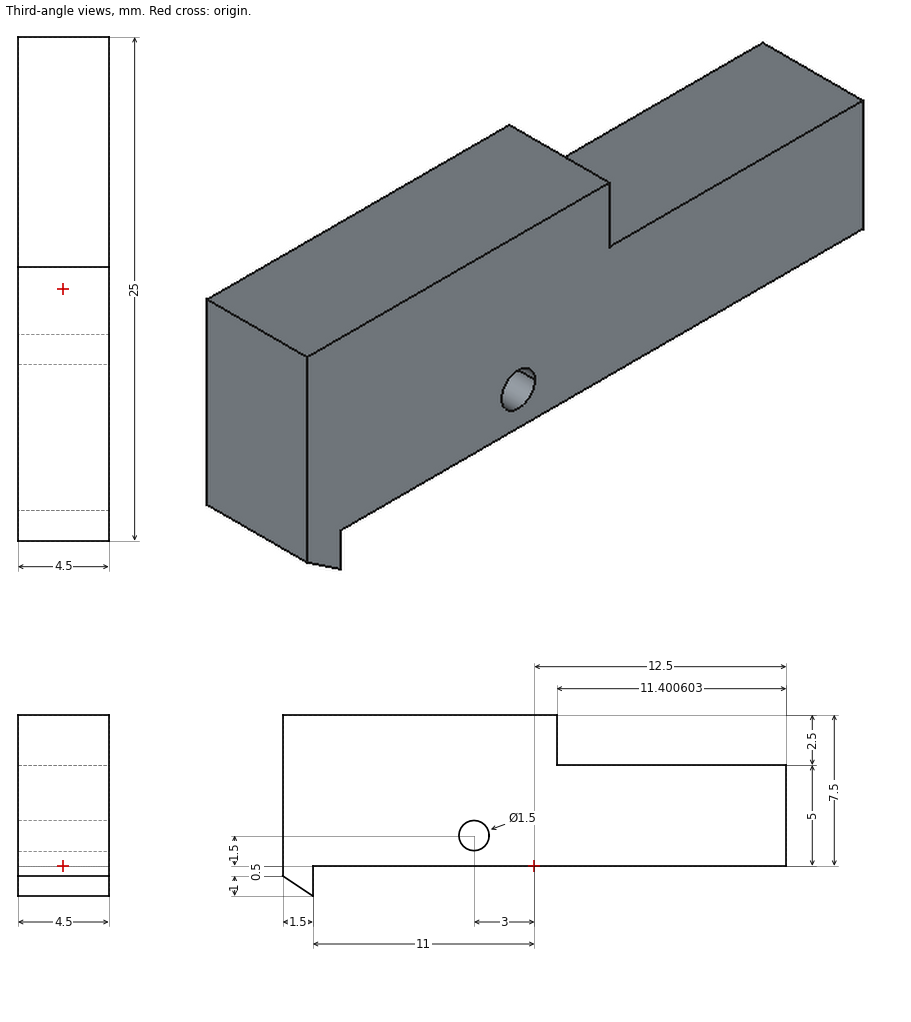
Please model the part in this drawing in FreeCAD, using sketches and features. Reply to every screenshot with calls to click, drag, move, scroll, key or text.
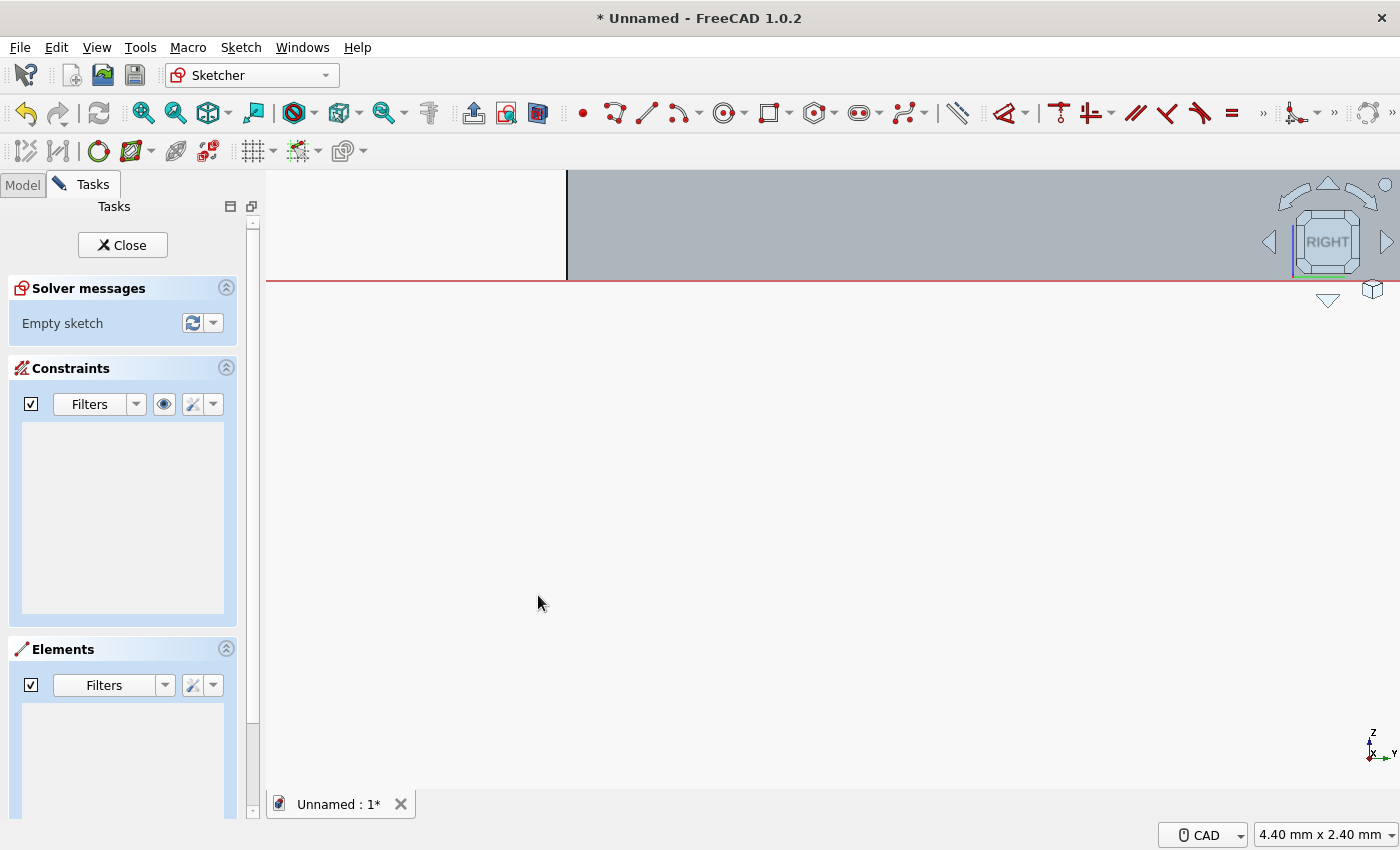
key(g)
key(m)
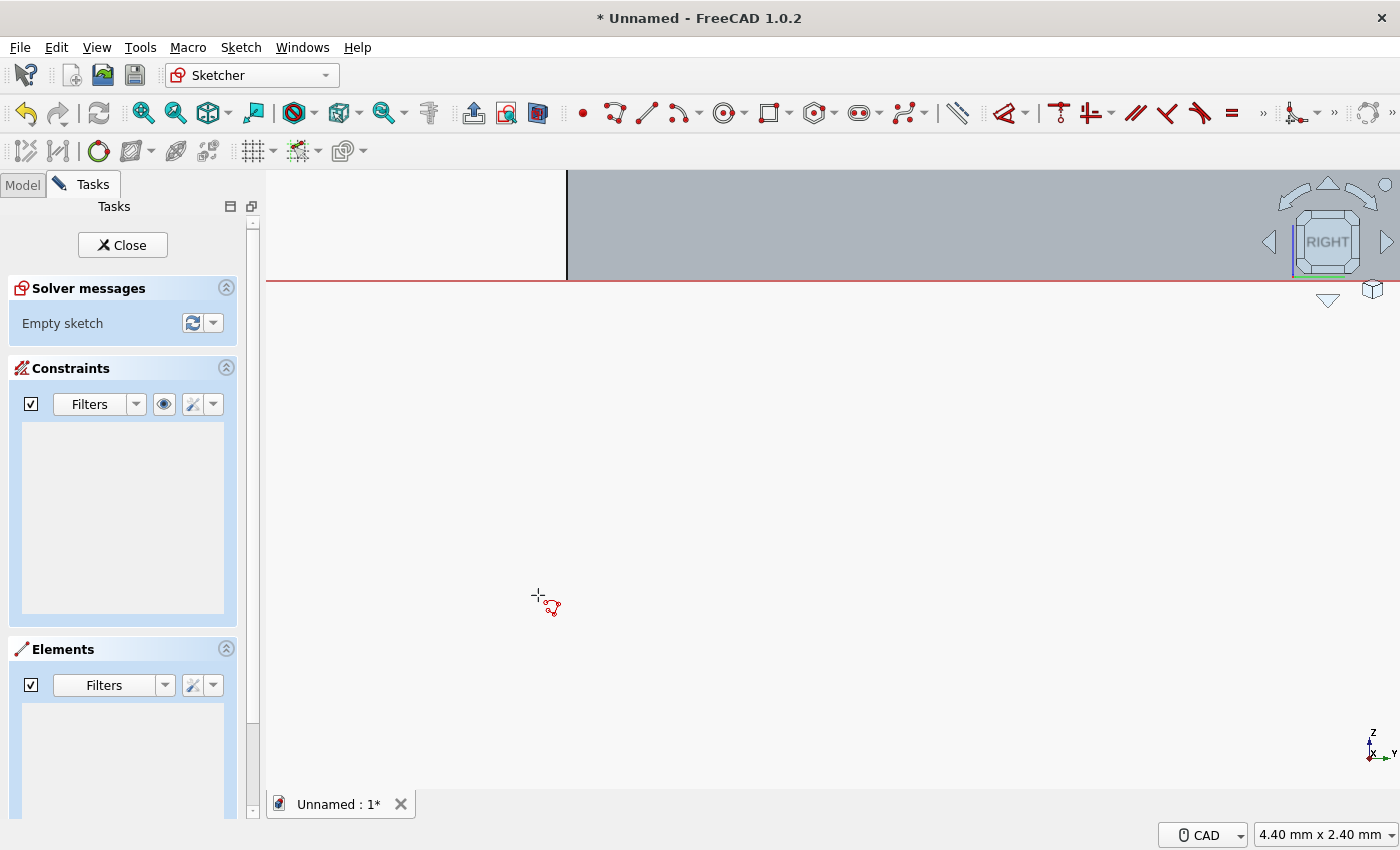
click(954, 281)
click(567, 290)
click(567, 410)
click(954, 667)
click(954, 281)
key(Escape)
key(Escape)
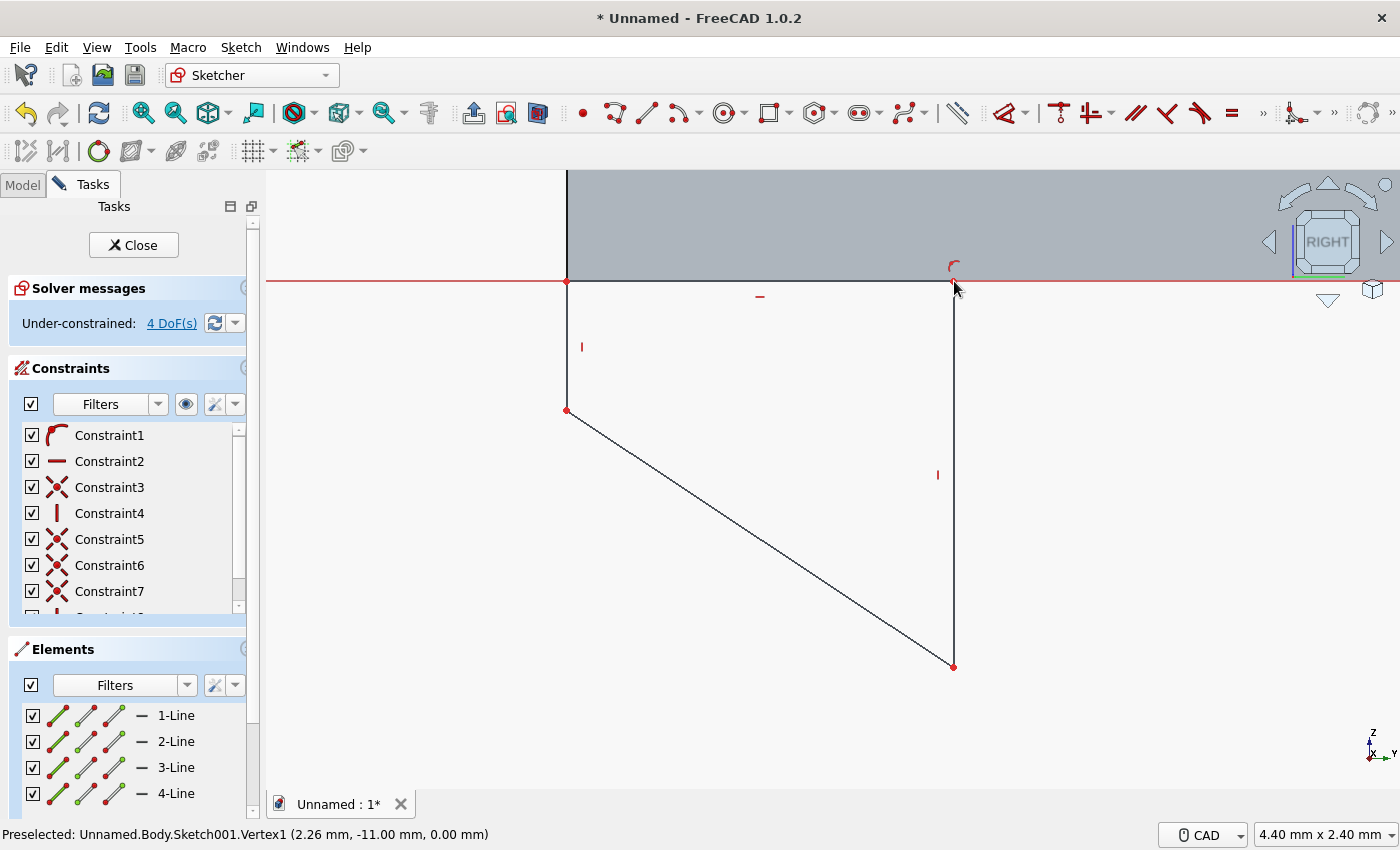
click(683, 488)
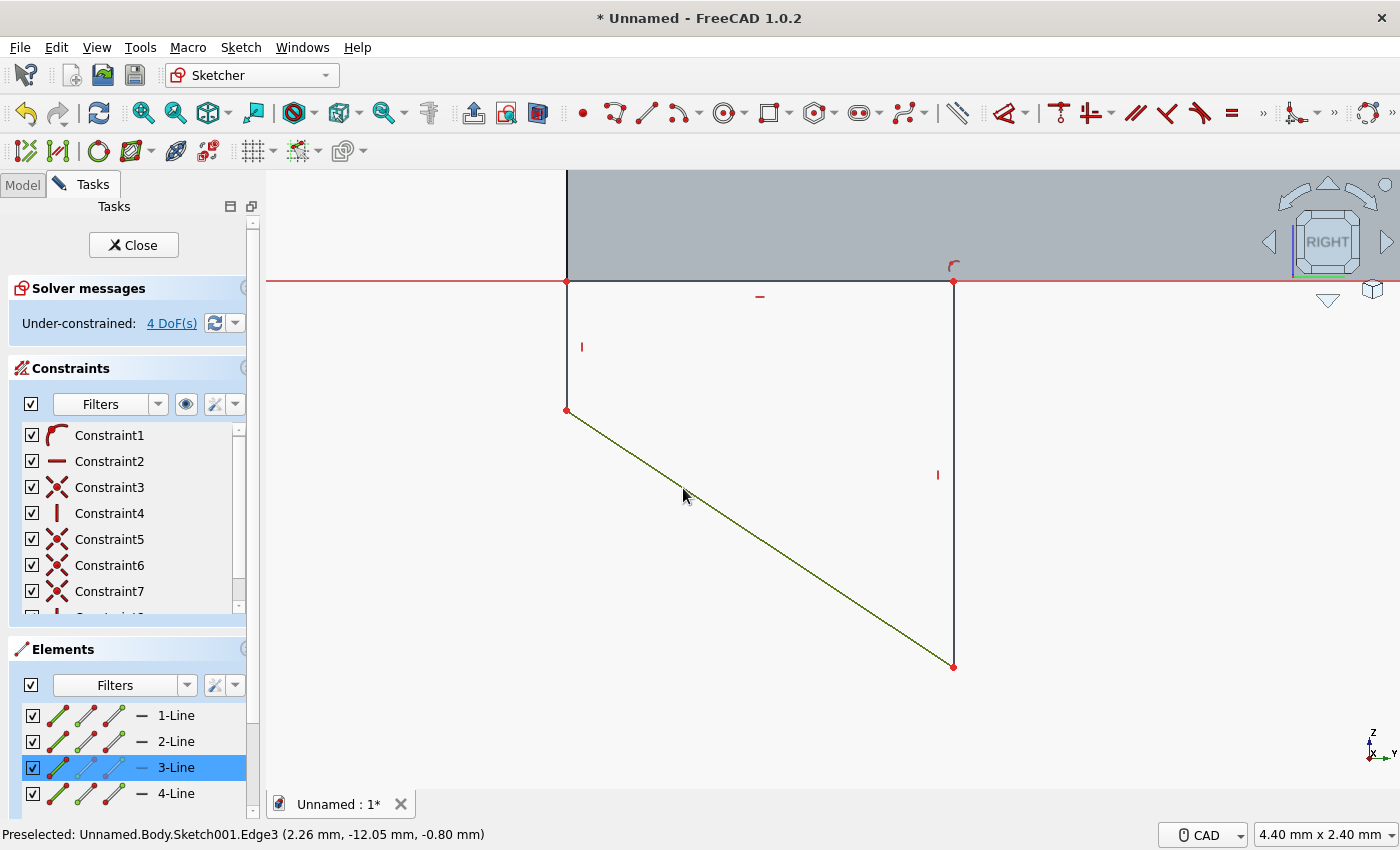
click(1028, 114)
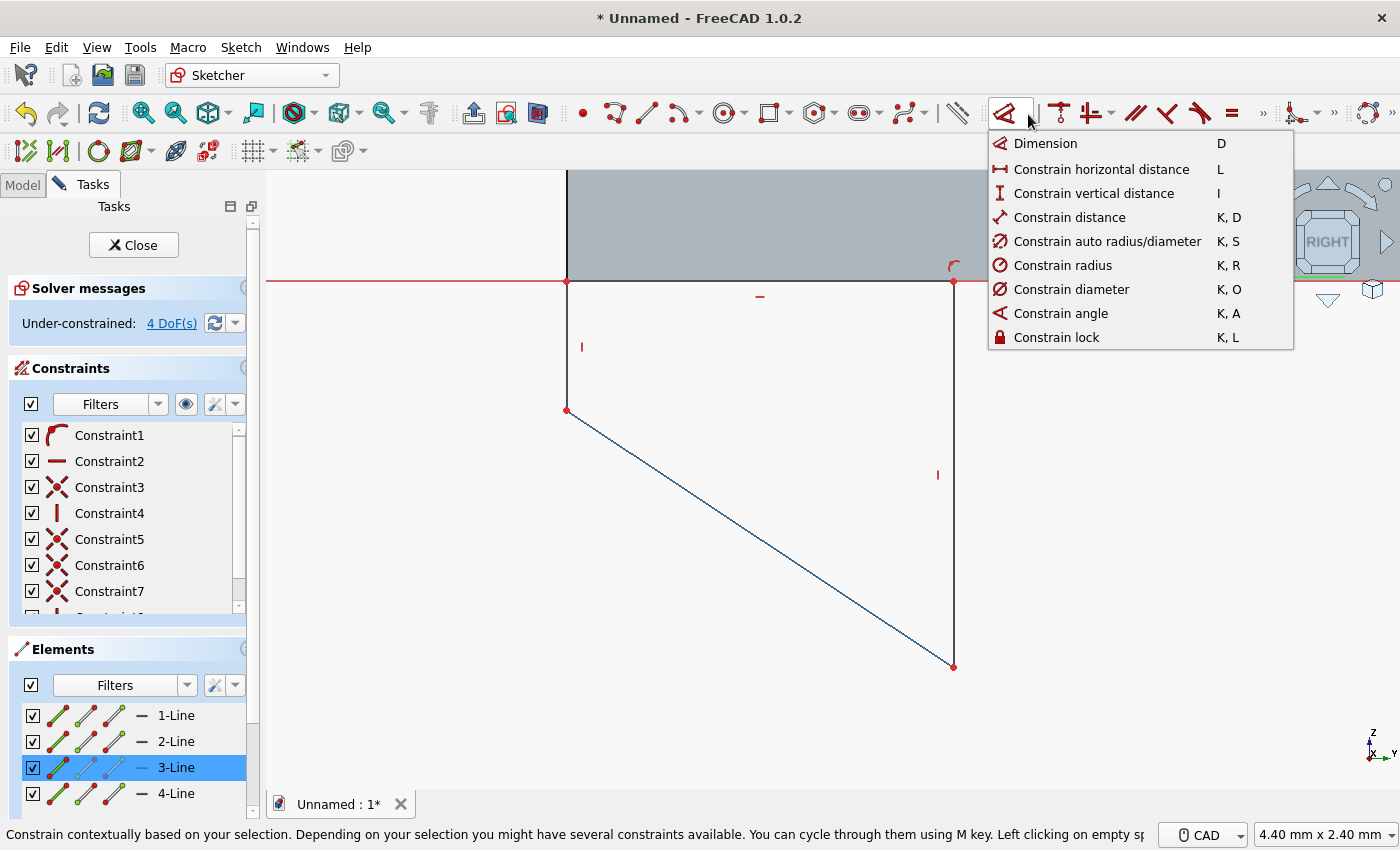
click(1141, 193)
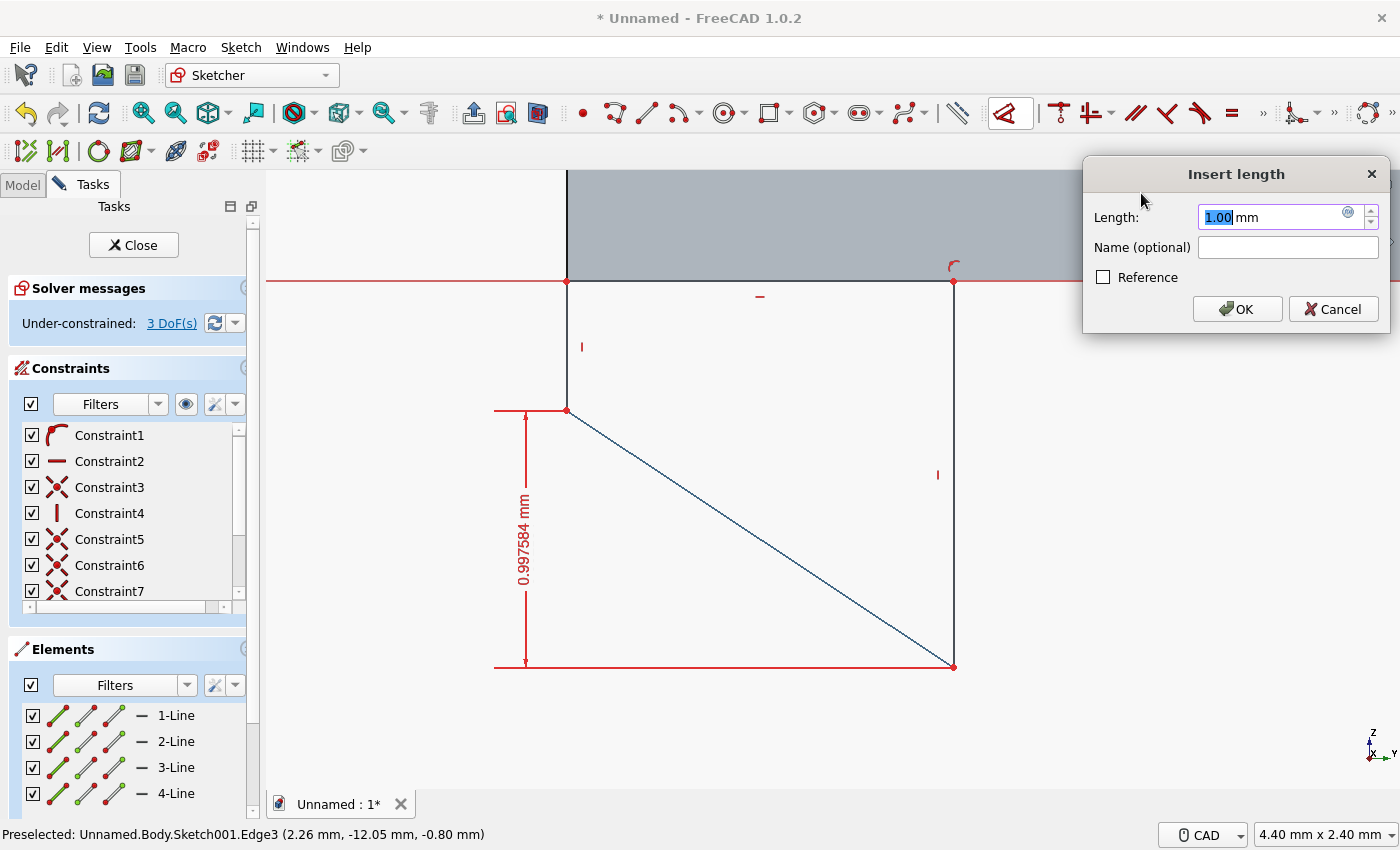
text(1)
key(Return)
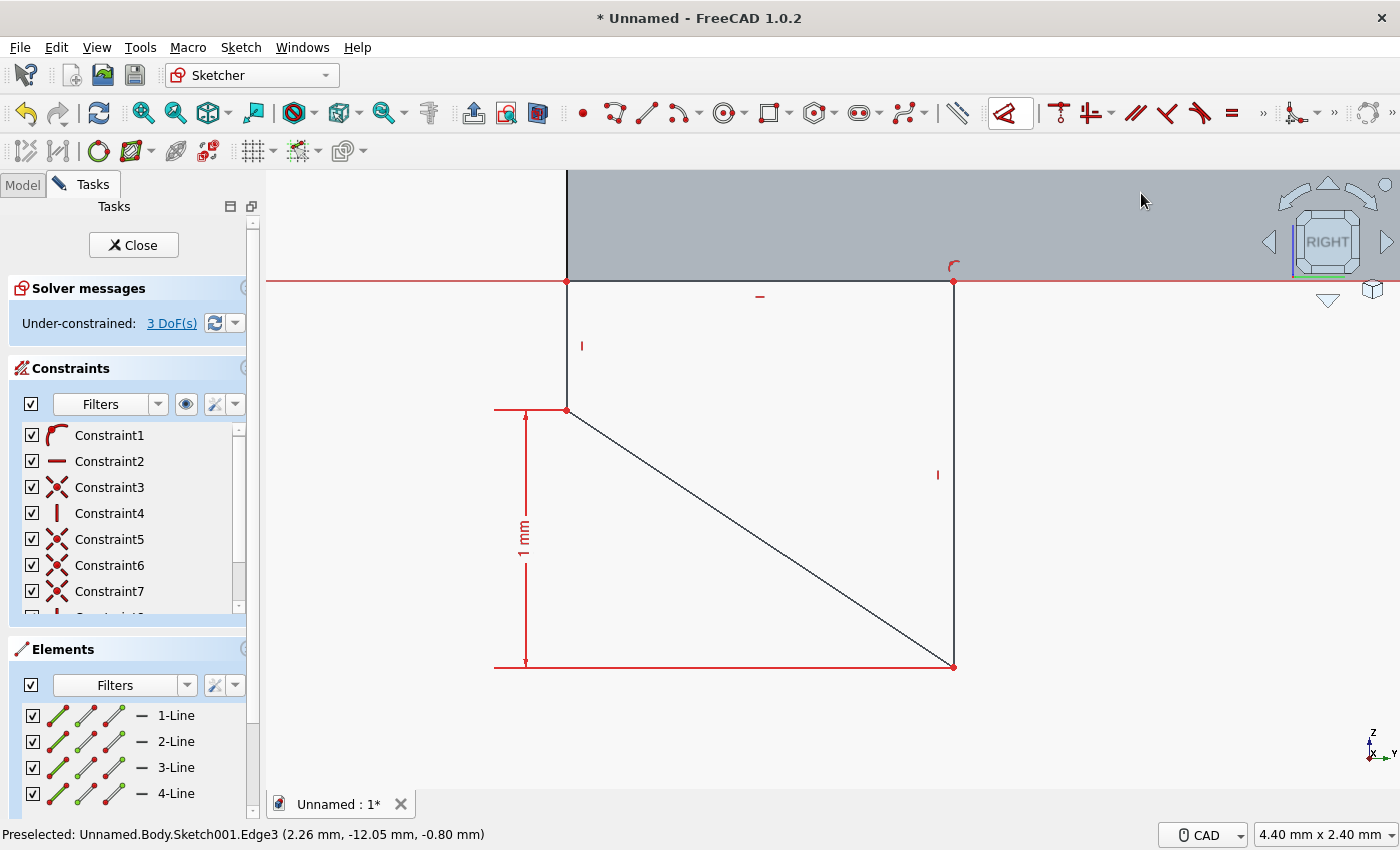
click(838, 281)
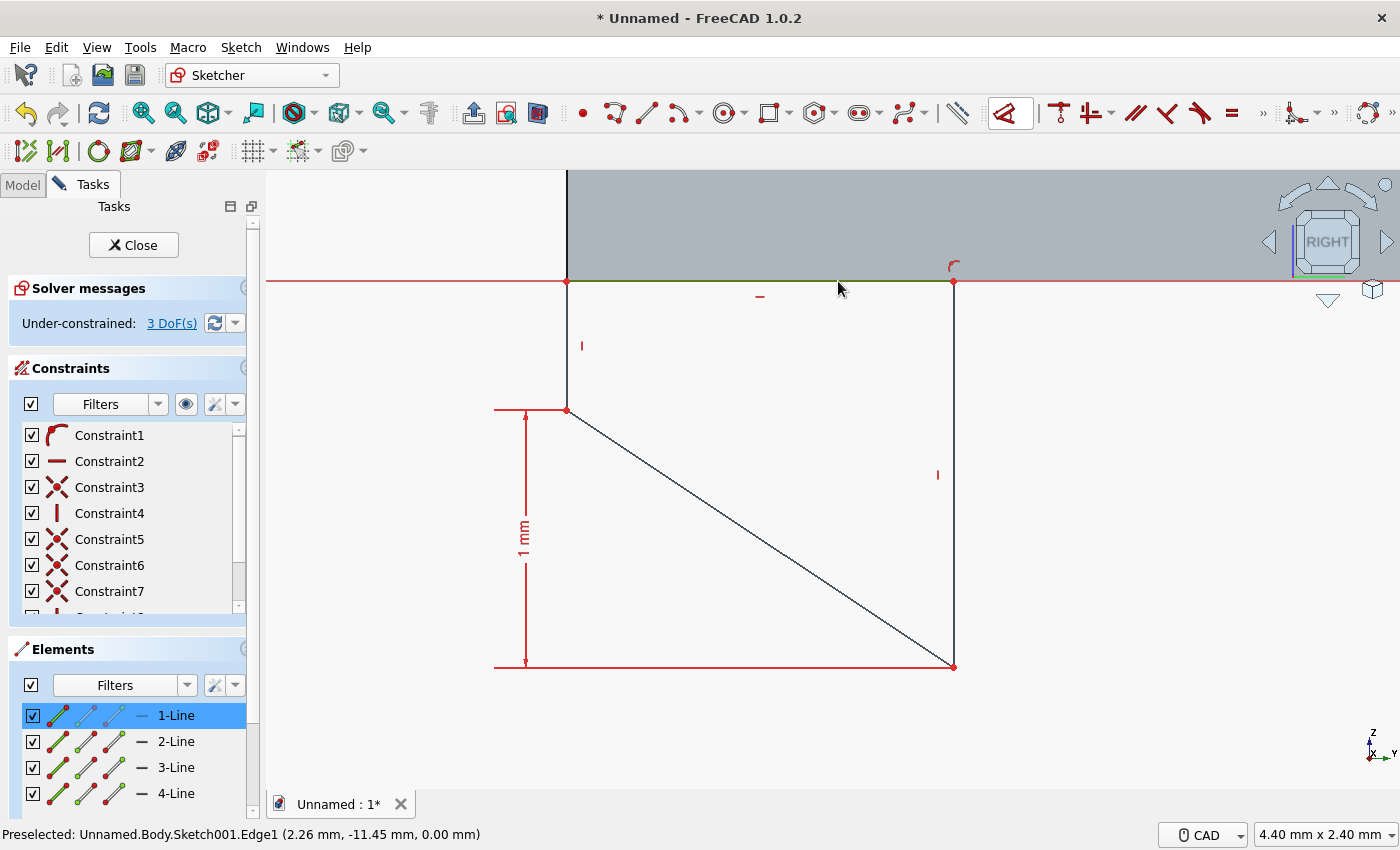
key(l)